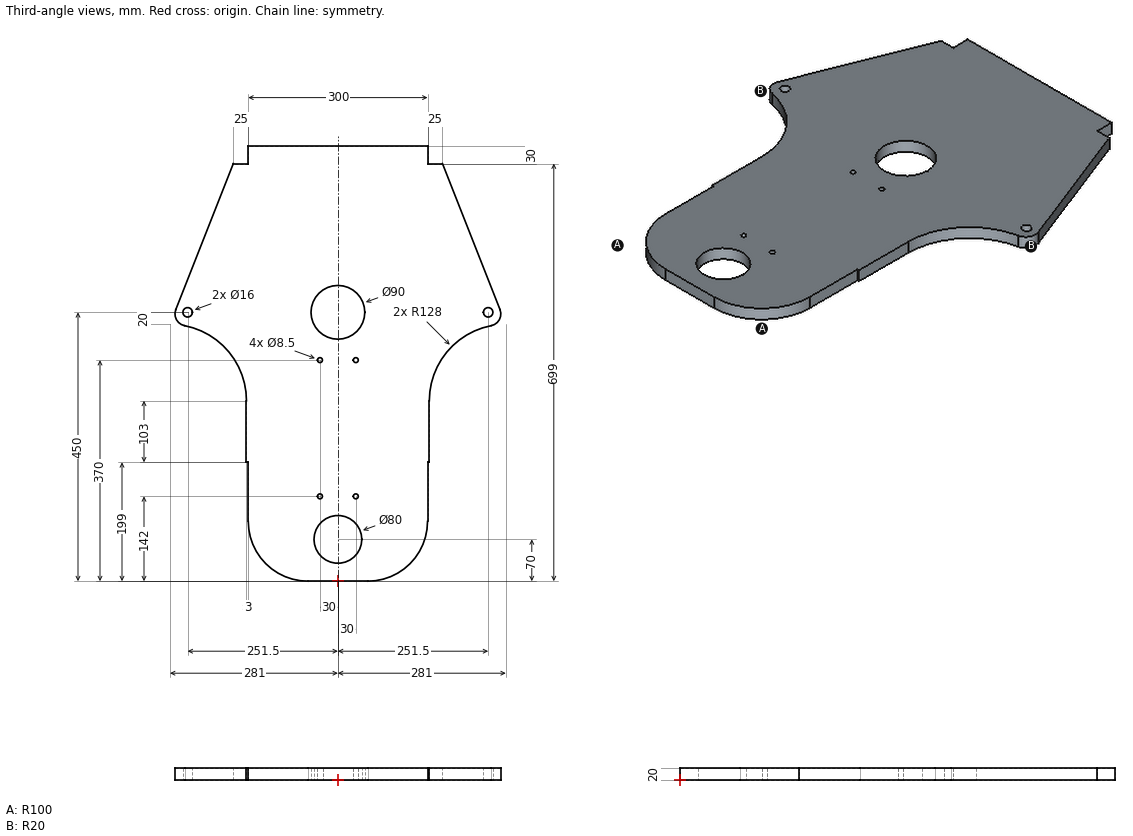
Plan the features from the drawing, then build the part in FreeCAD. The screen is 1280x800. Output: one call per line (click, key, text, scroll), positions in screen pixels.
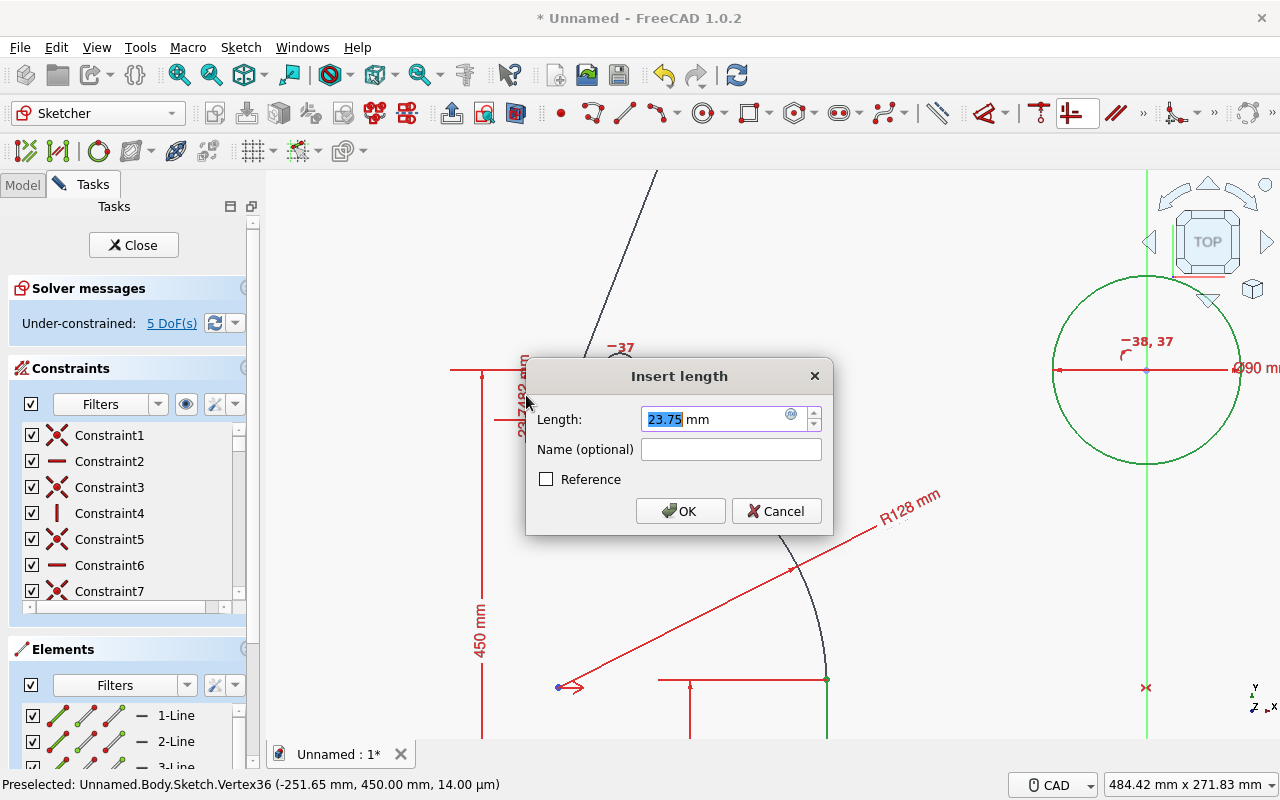
text(20)
key(Return)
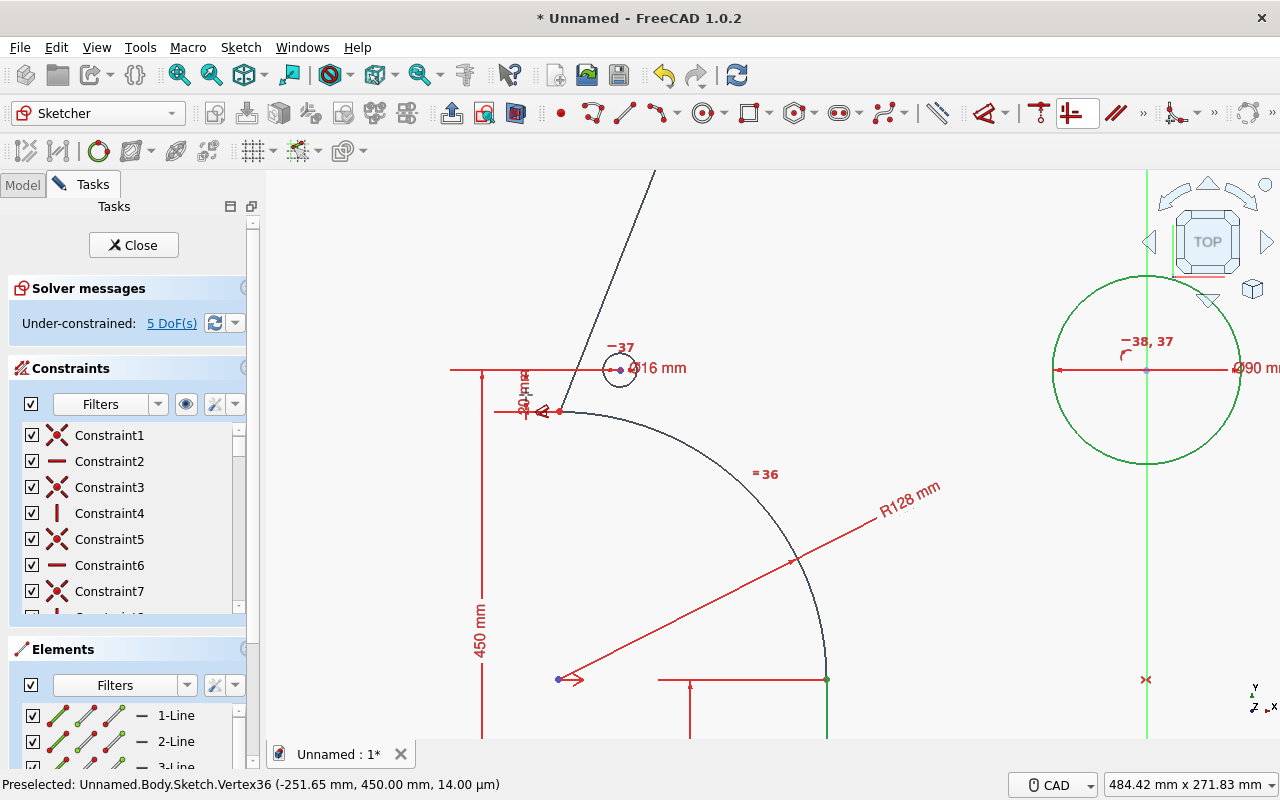
scroll(560, 424, down, 7)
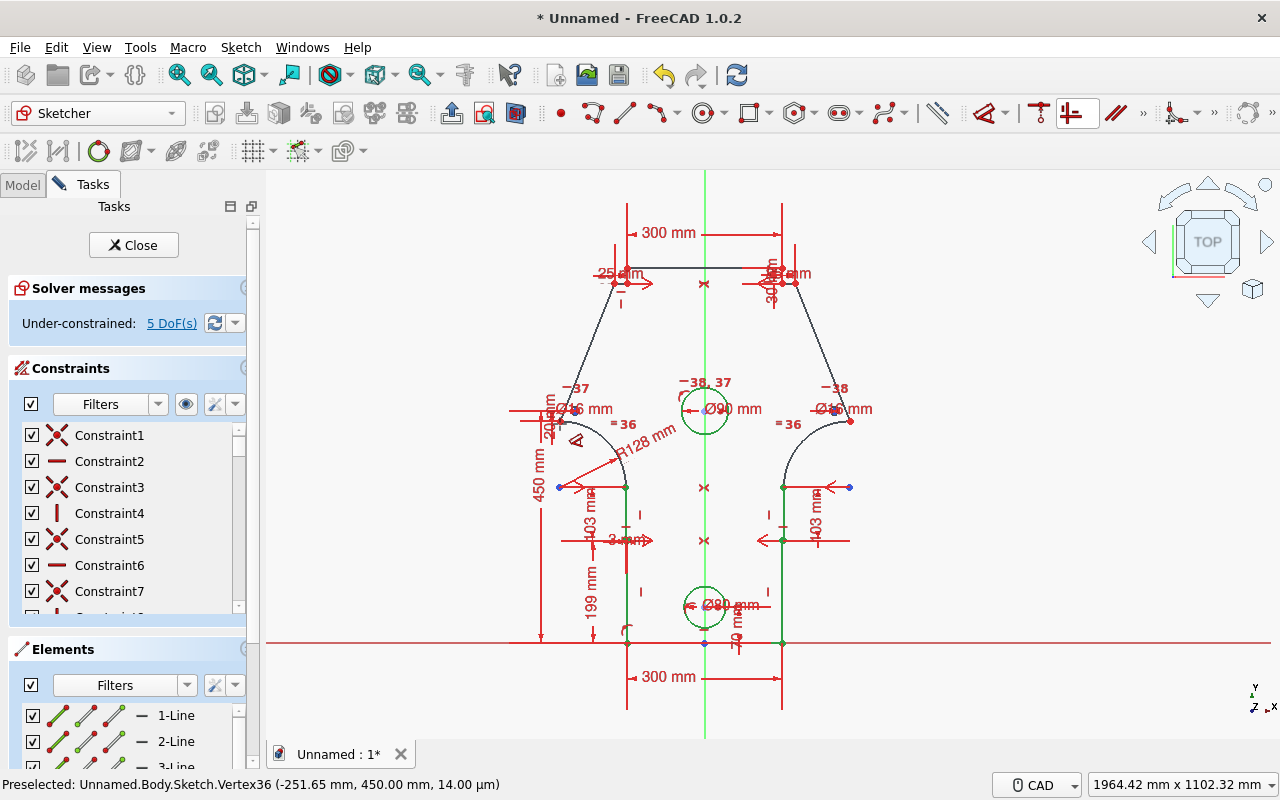
click(850, 421)
click(778, 677)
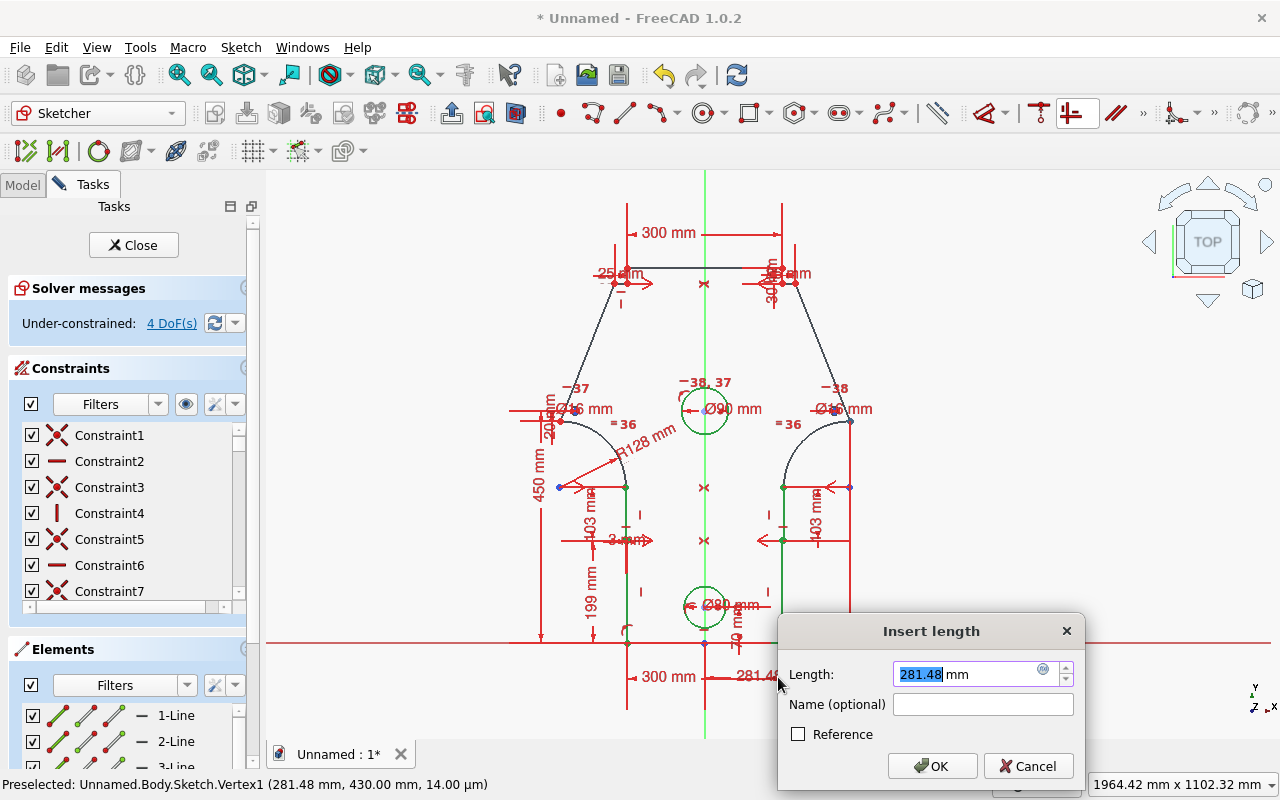
text(281)
key(Return)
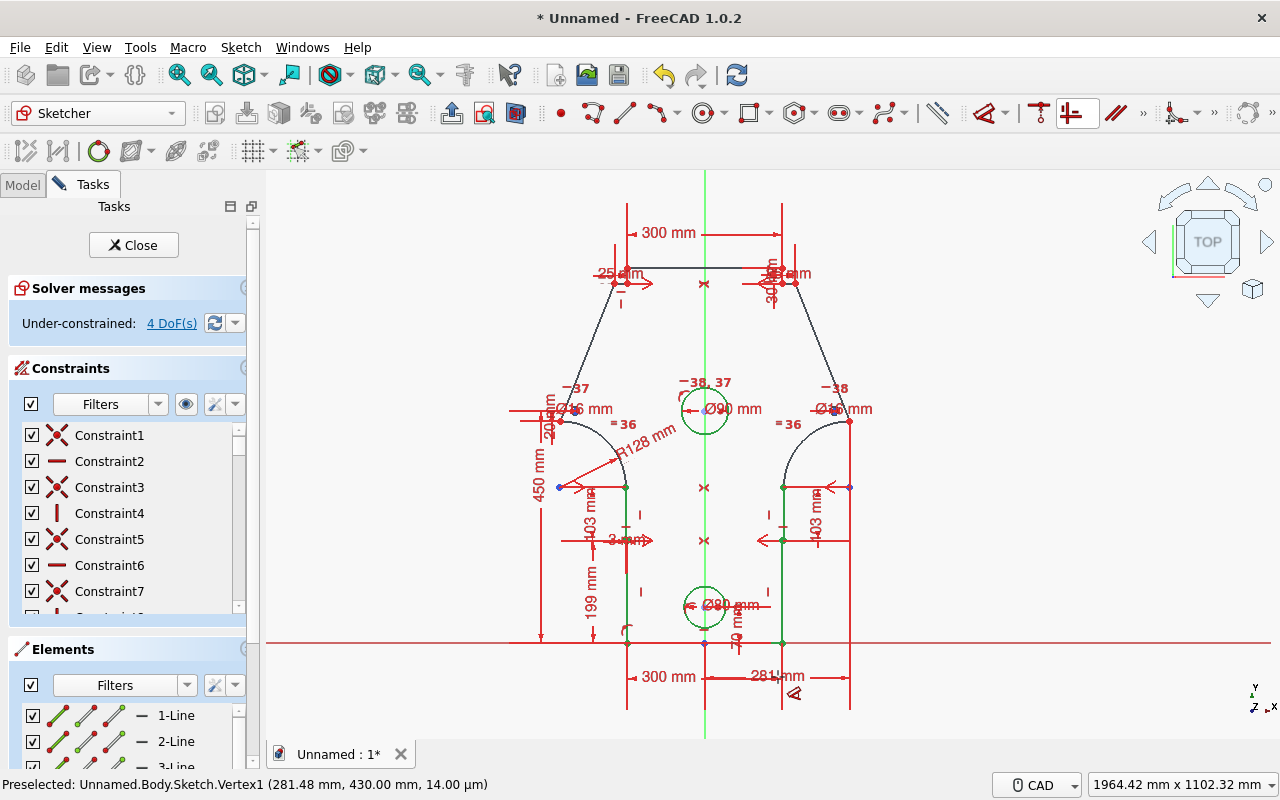
click(795, 284)
click(829, 463)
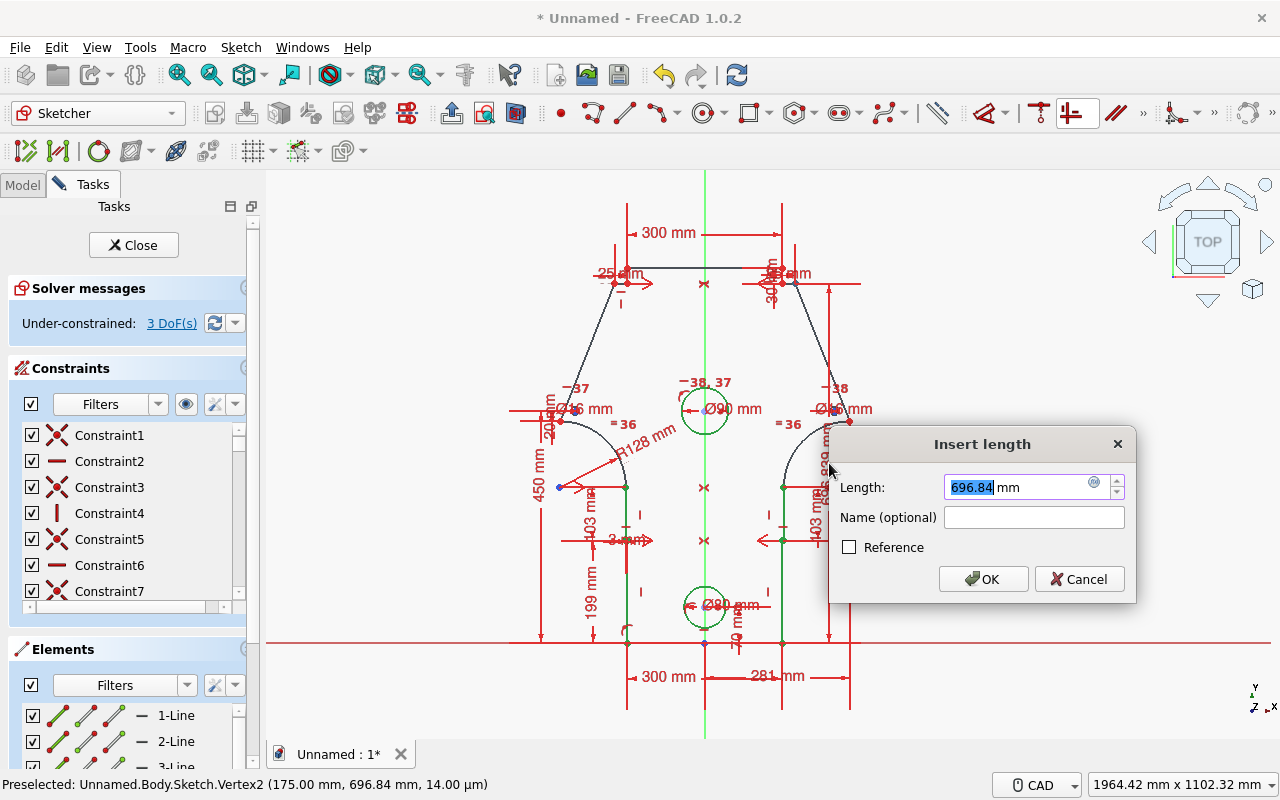
text(699)
key(Return)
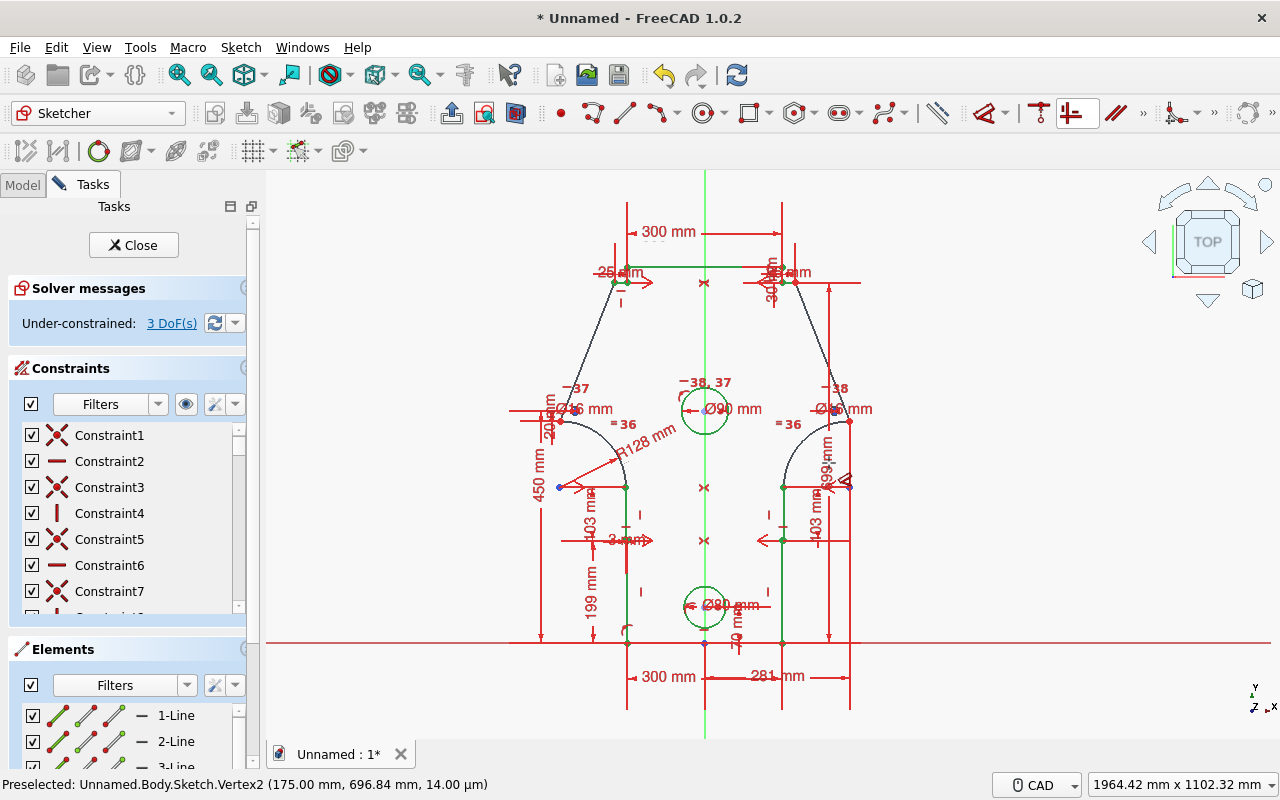
click(560, 421)
click(582, 677)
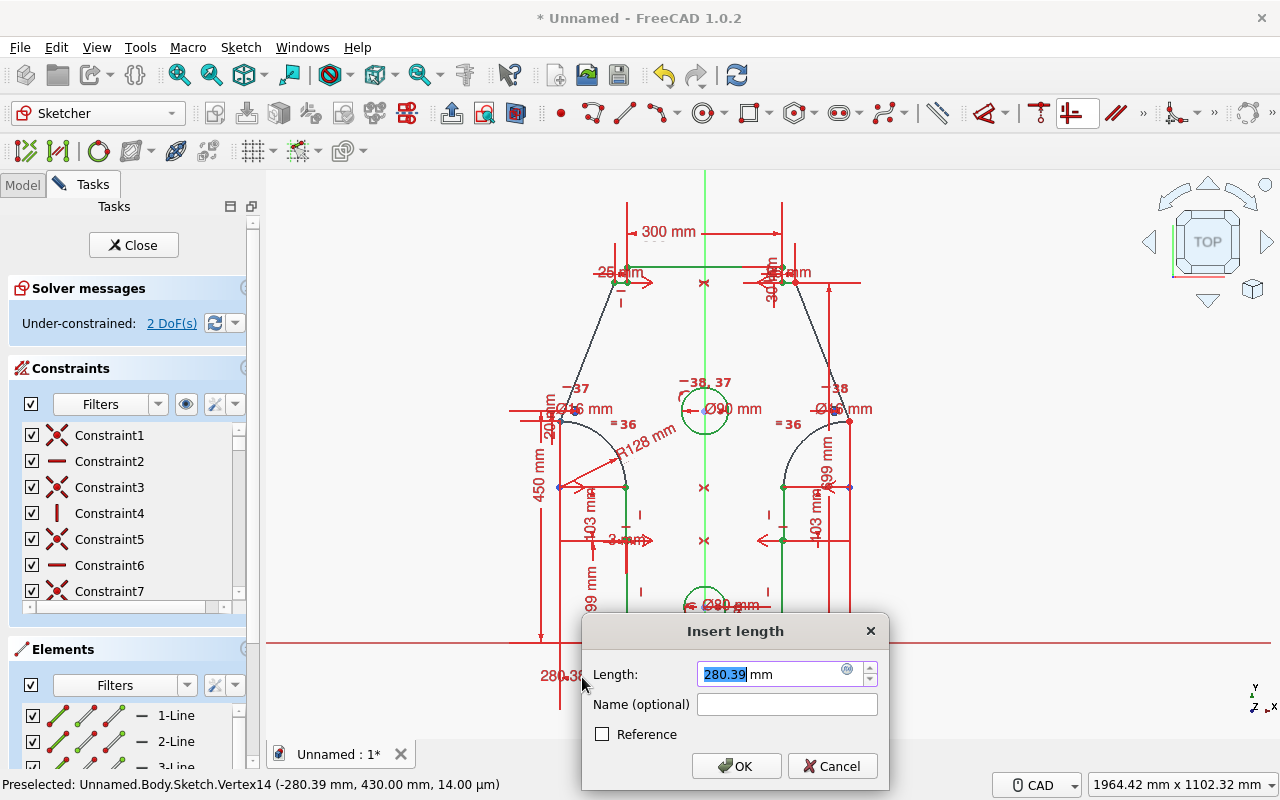
text(281)
key(Return)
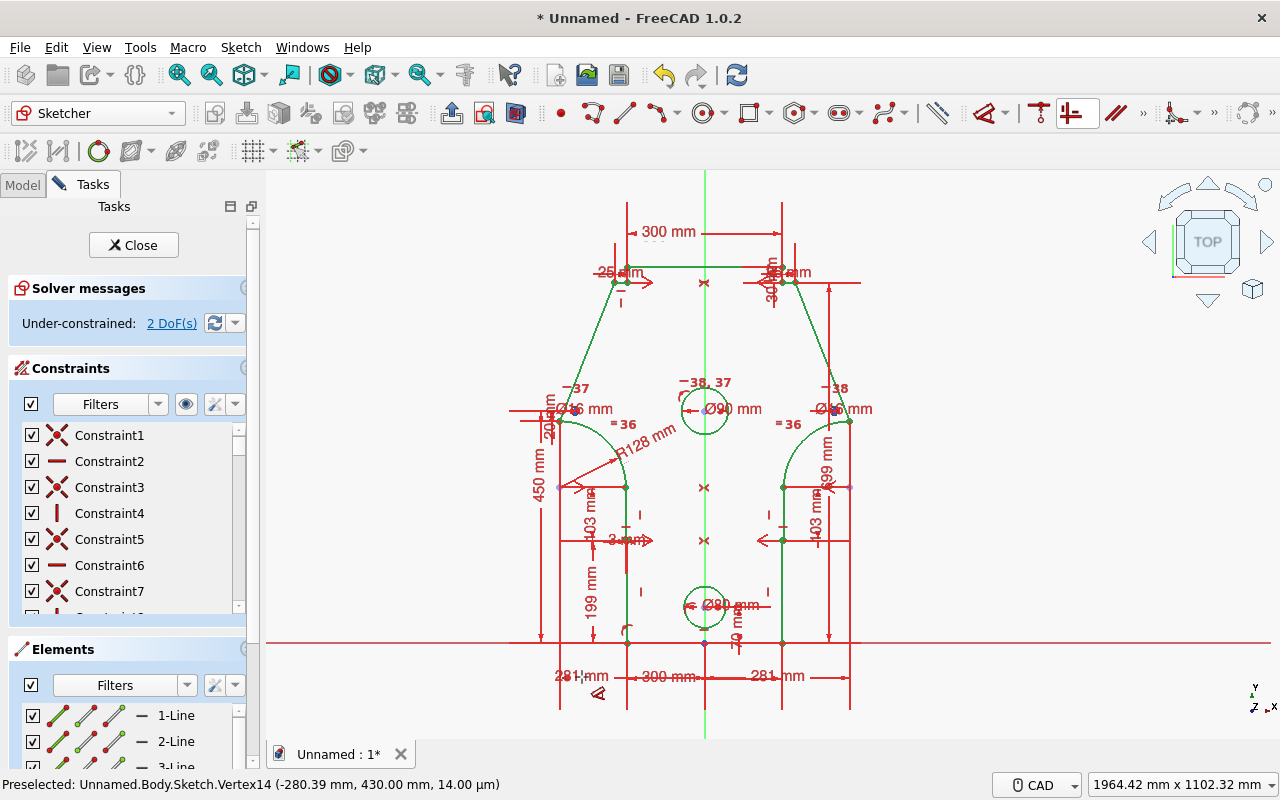
click(575, 411)
click(640, 377)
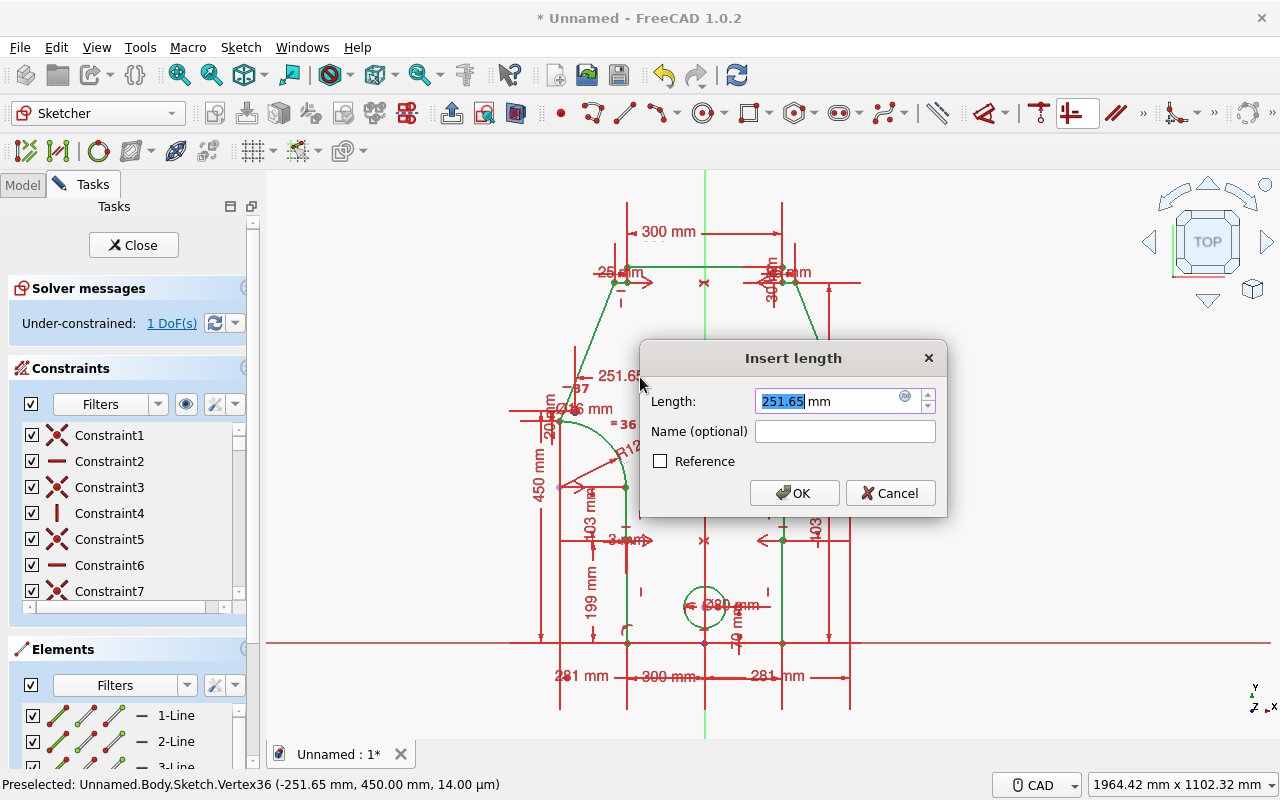
text(251.5)
key(Return)